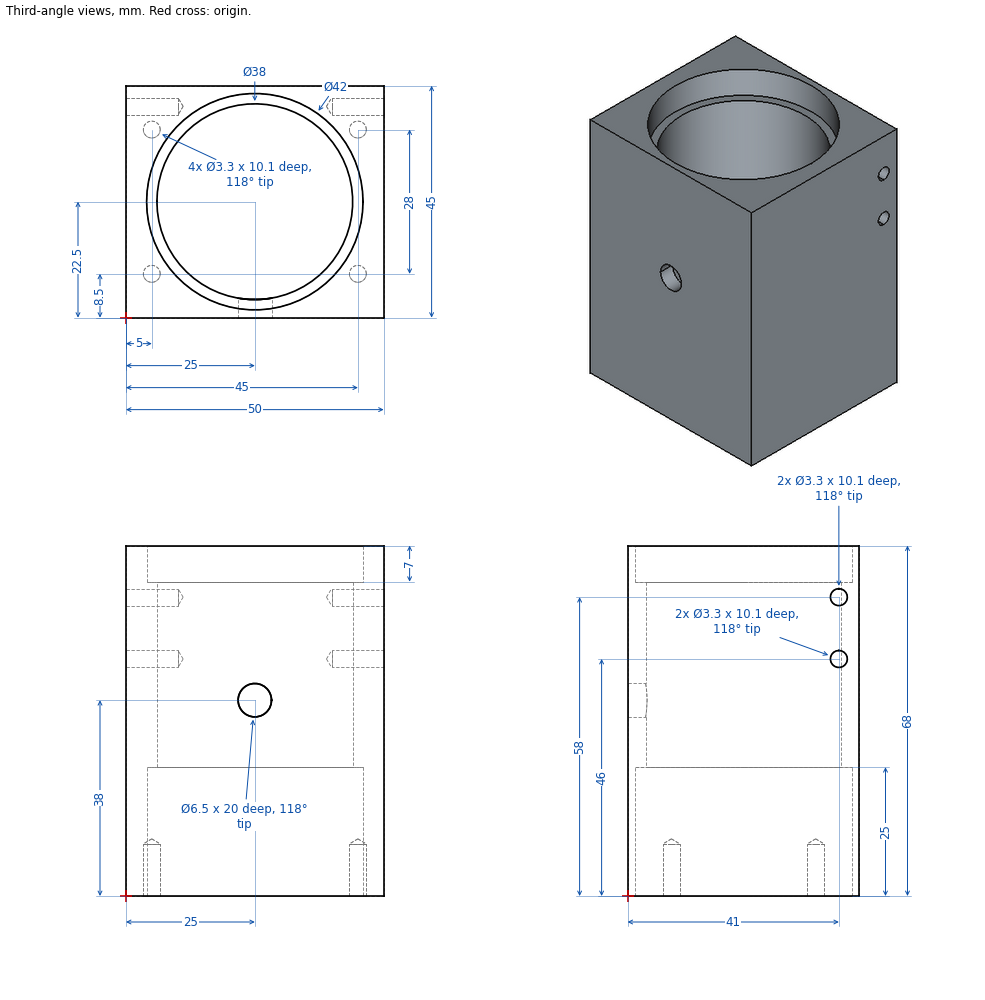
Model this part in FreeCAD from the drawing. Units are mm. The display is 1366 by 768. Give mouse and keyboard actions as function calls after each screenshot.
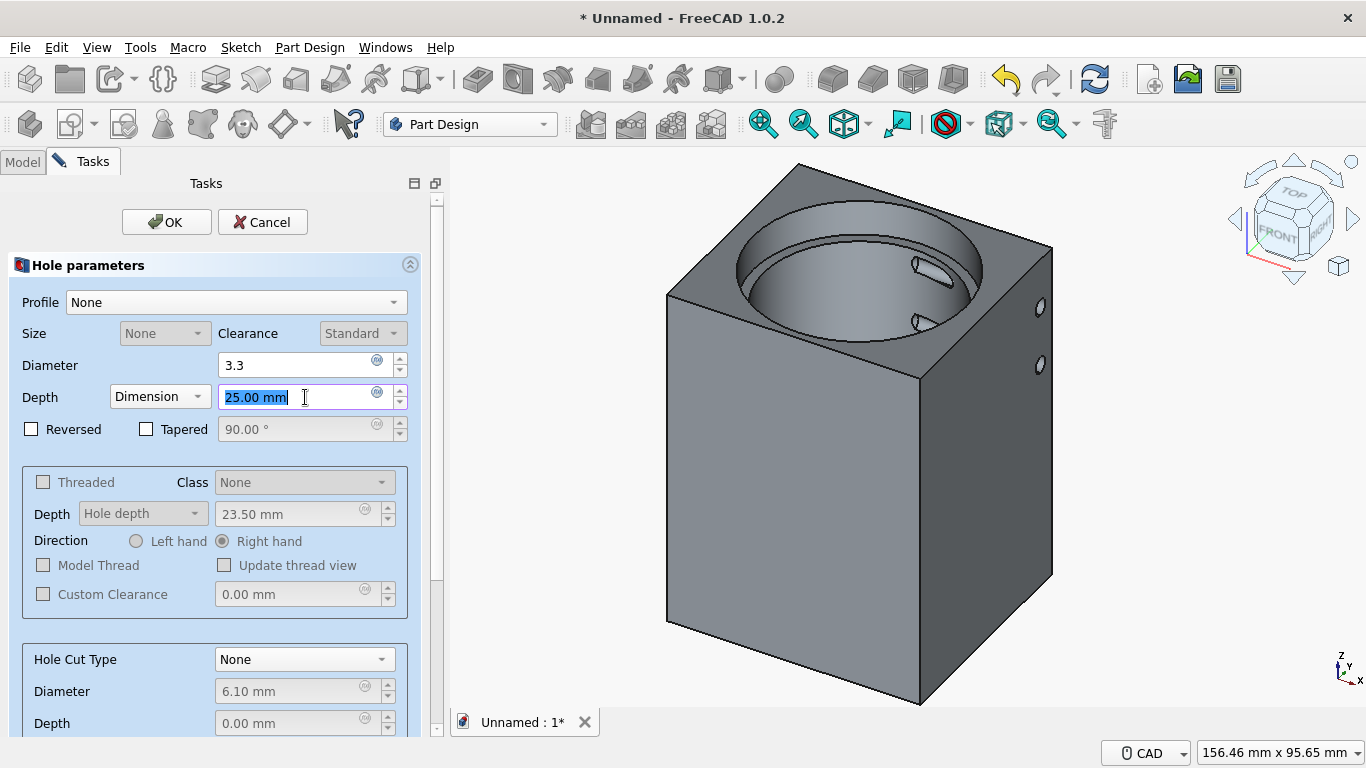
text(10.1)
key(Tab)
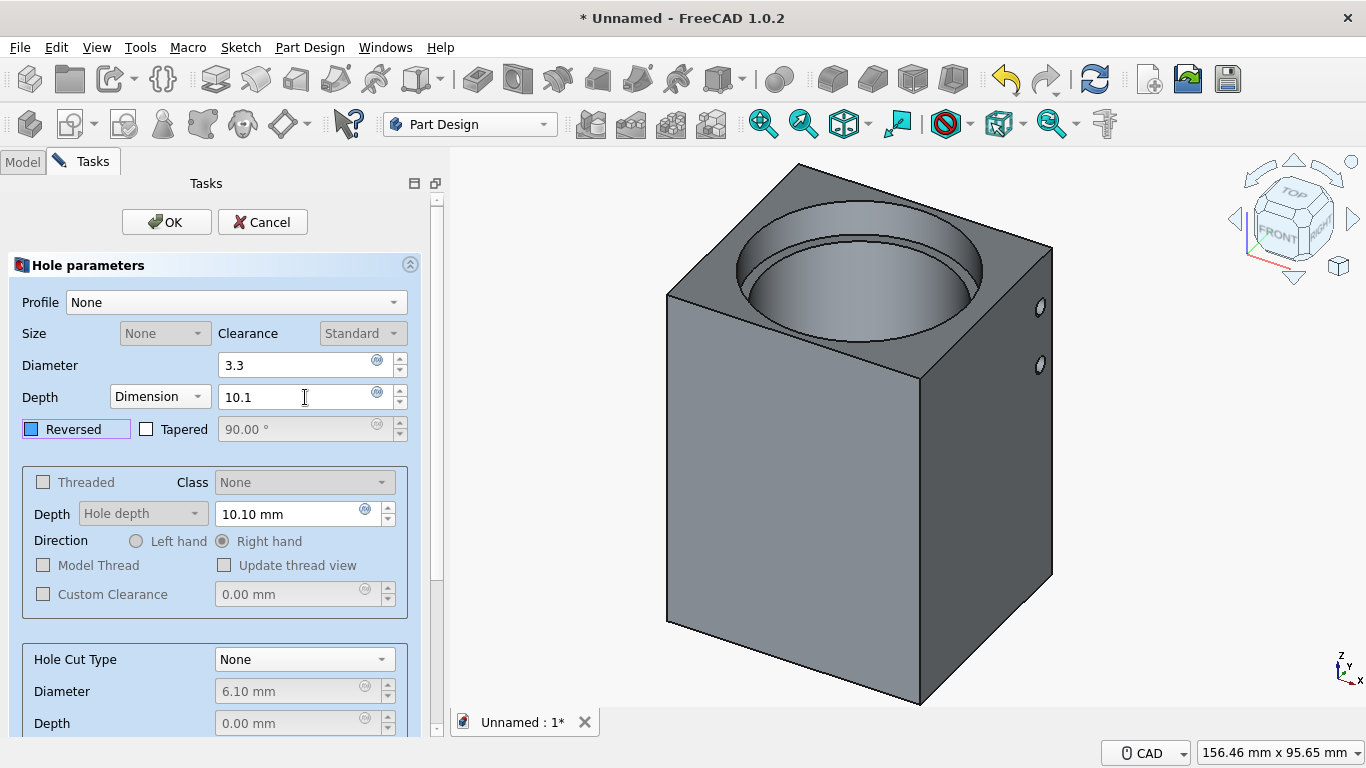
click(167, 222)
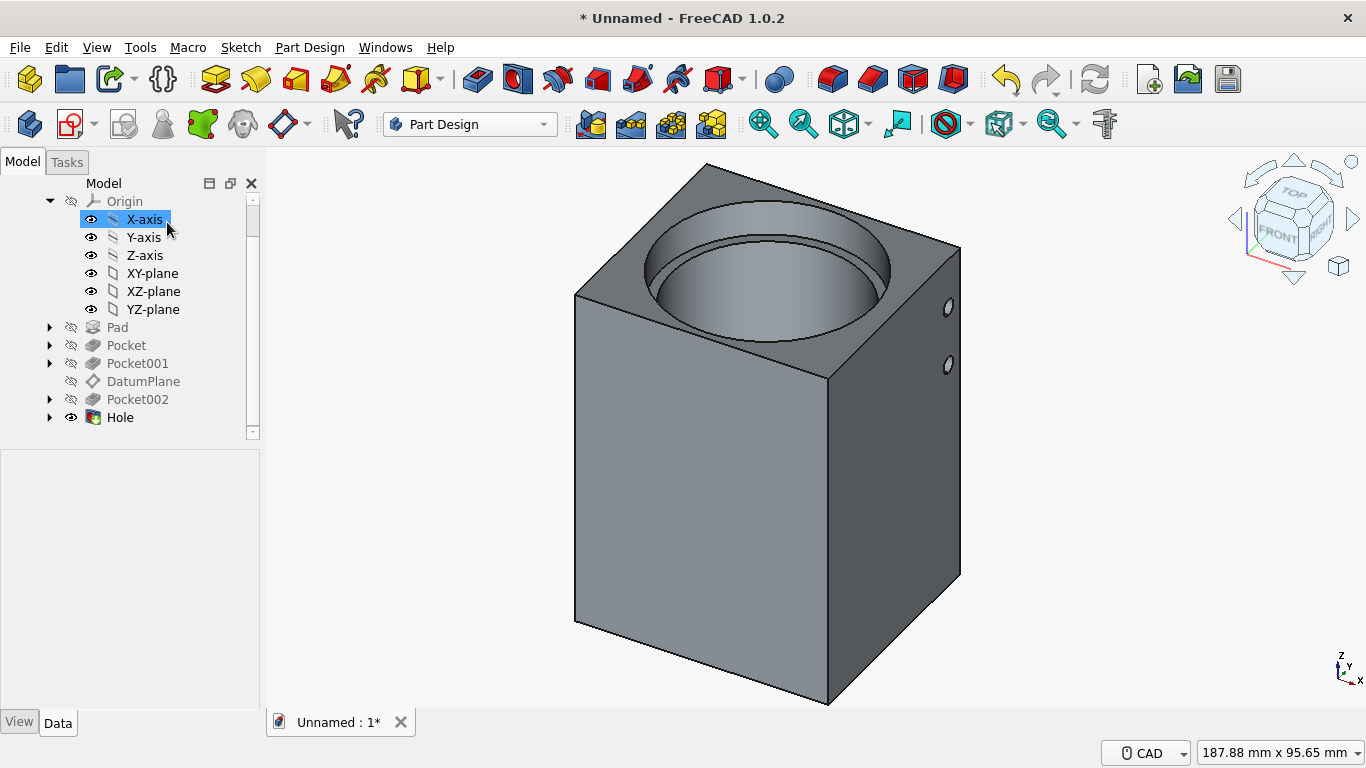
key(6)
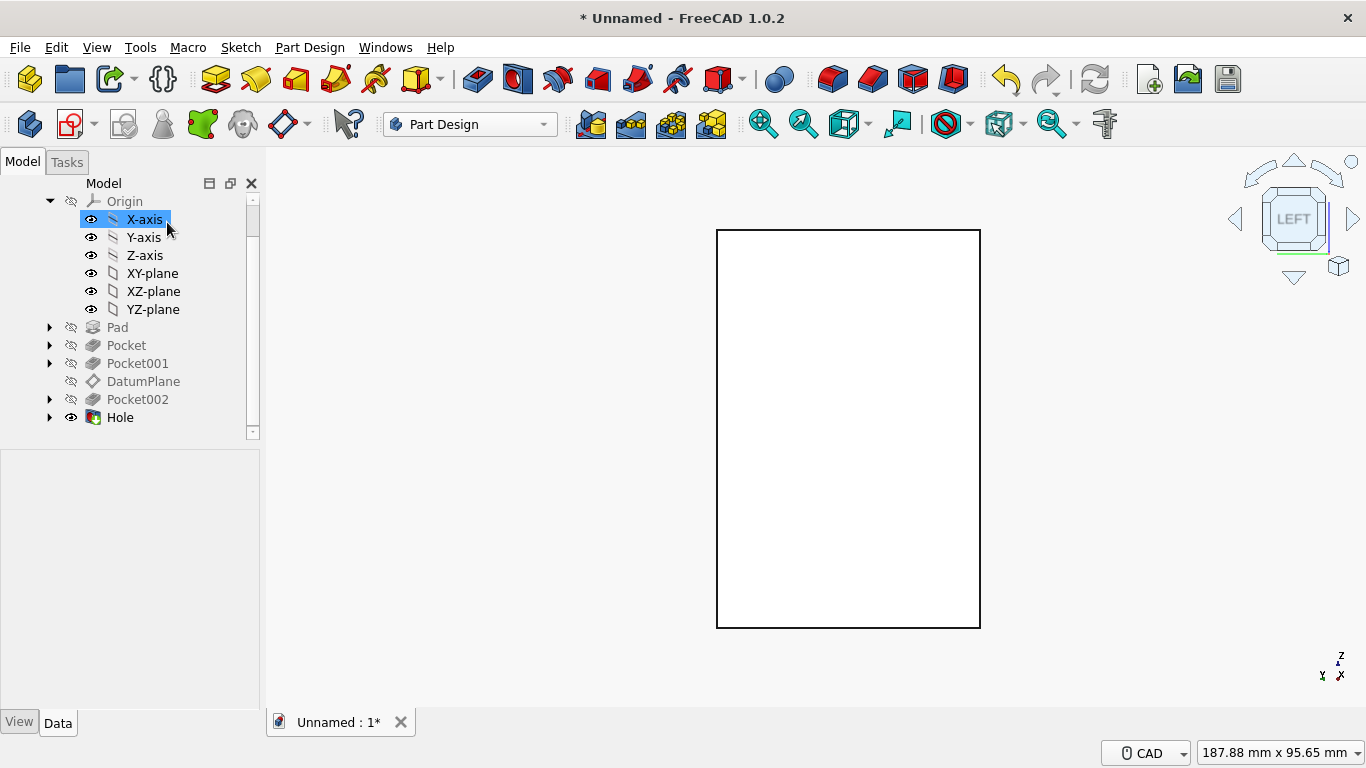
click(849, 372)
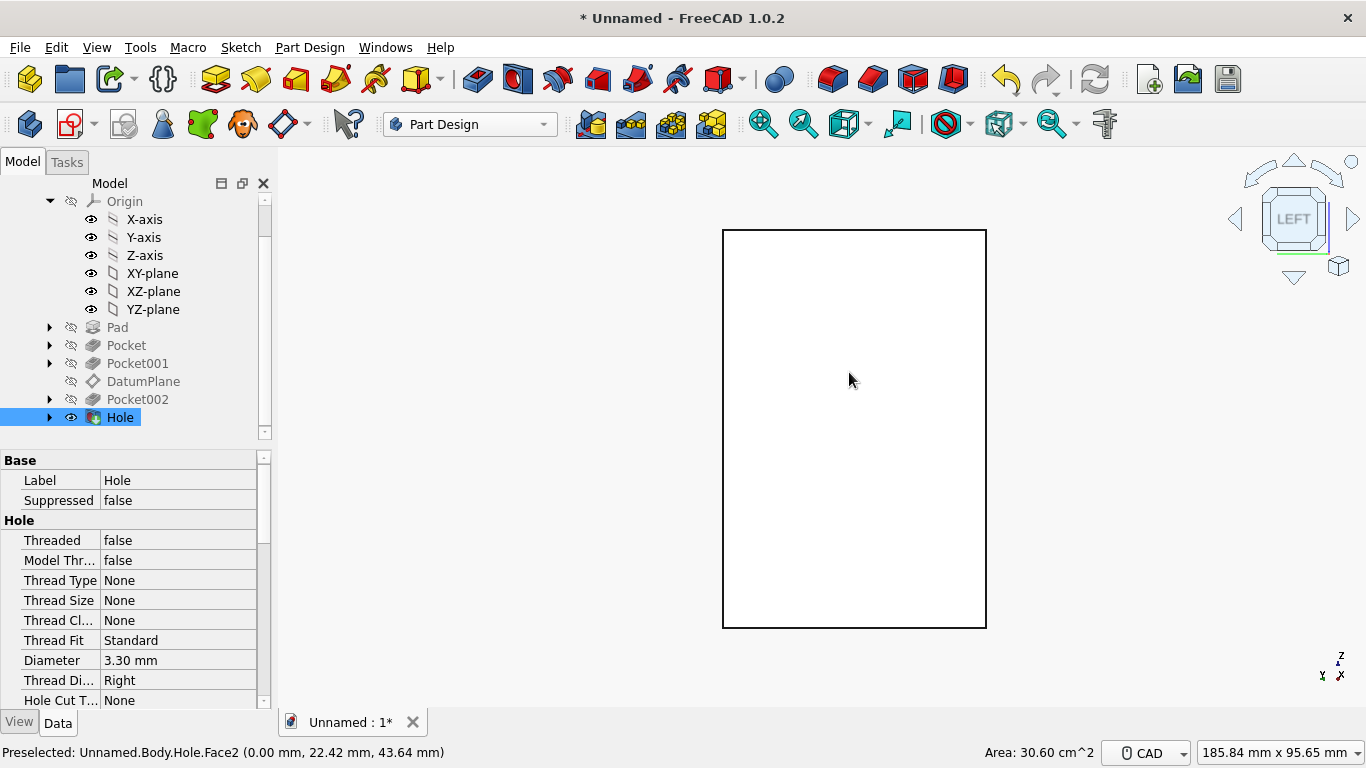
click(70, 124)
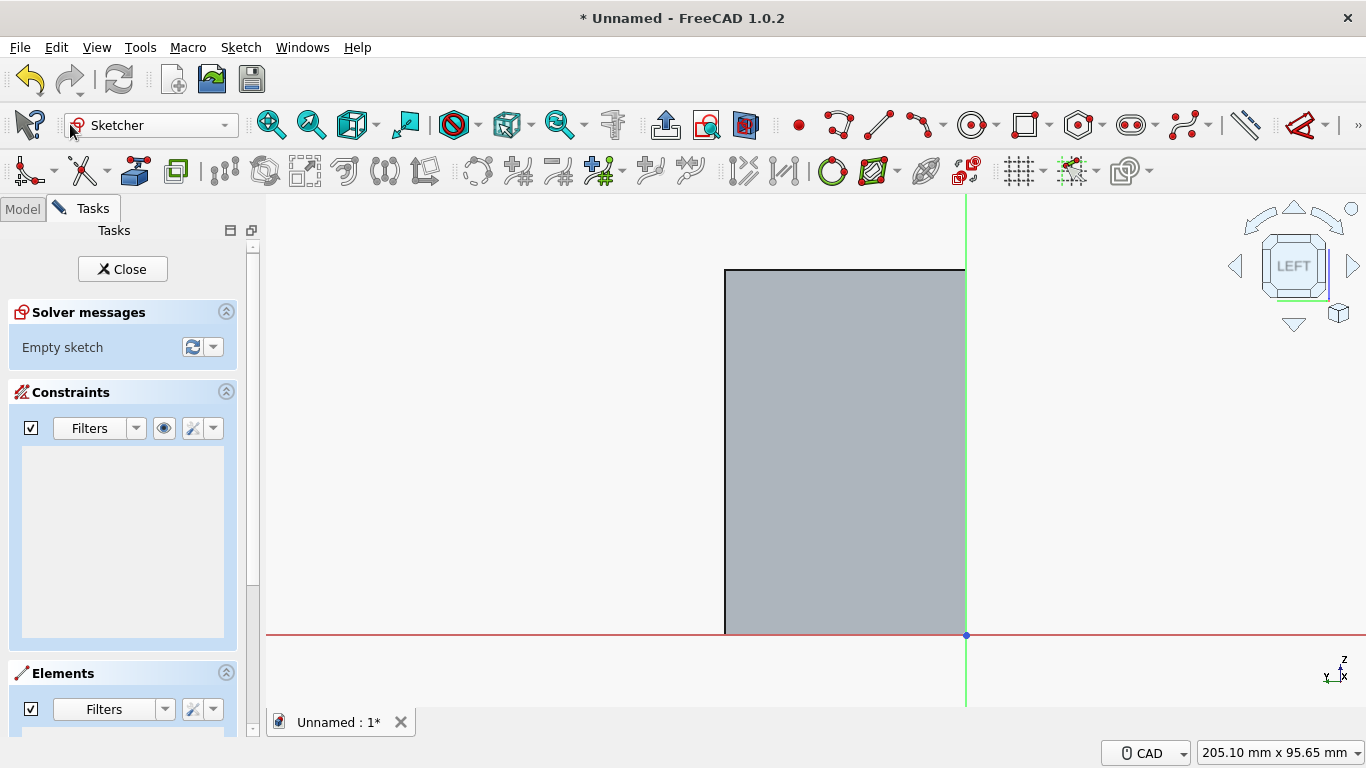
scroll(746, 325, up, 7)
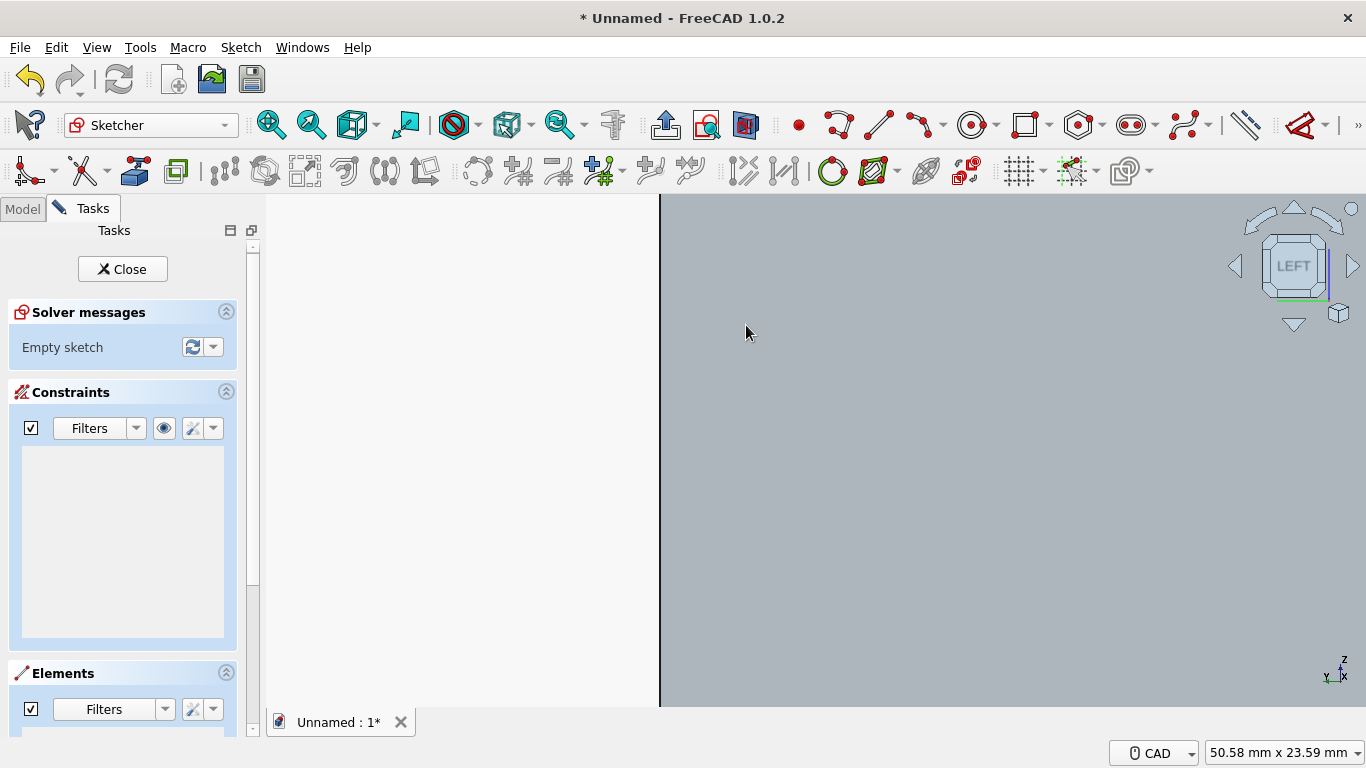
click(972, 126)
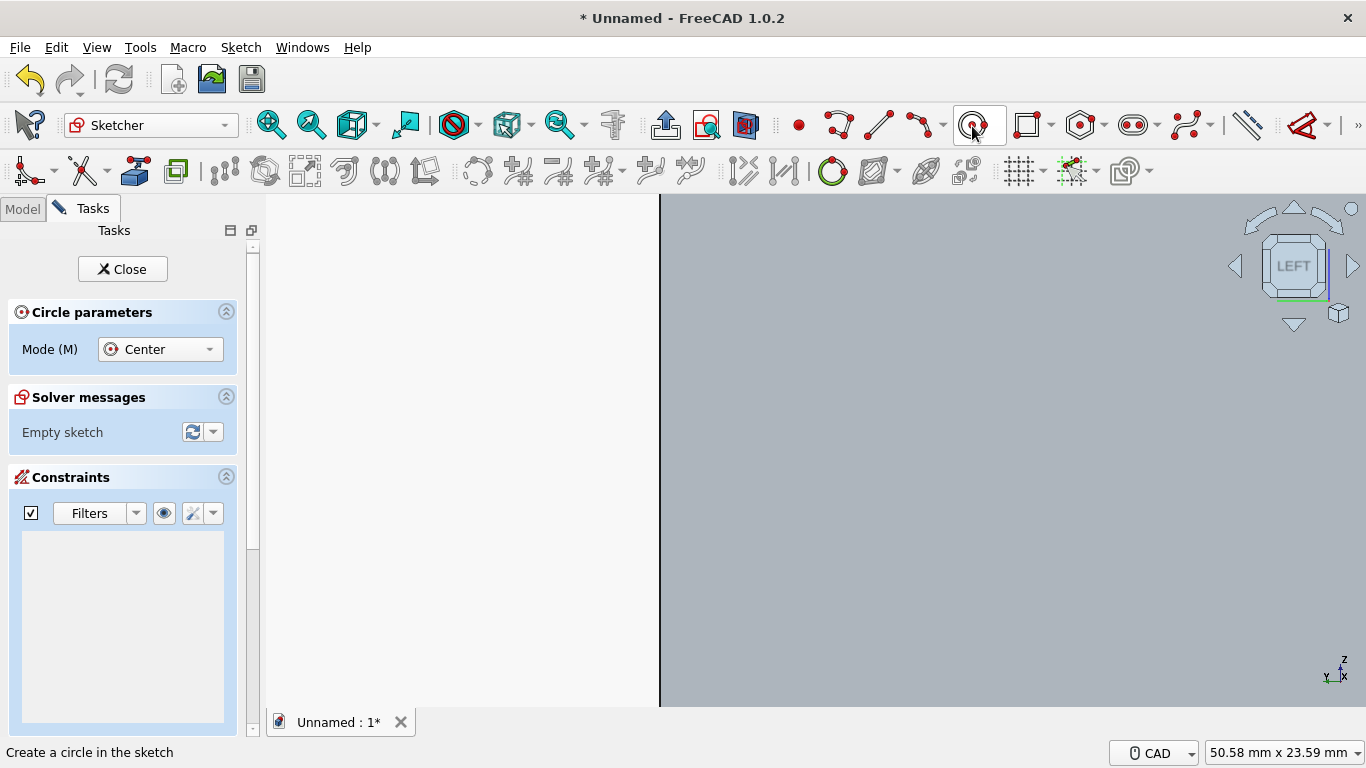
click(747, 581)
move(772, 556)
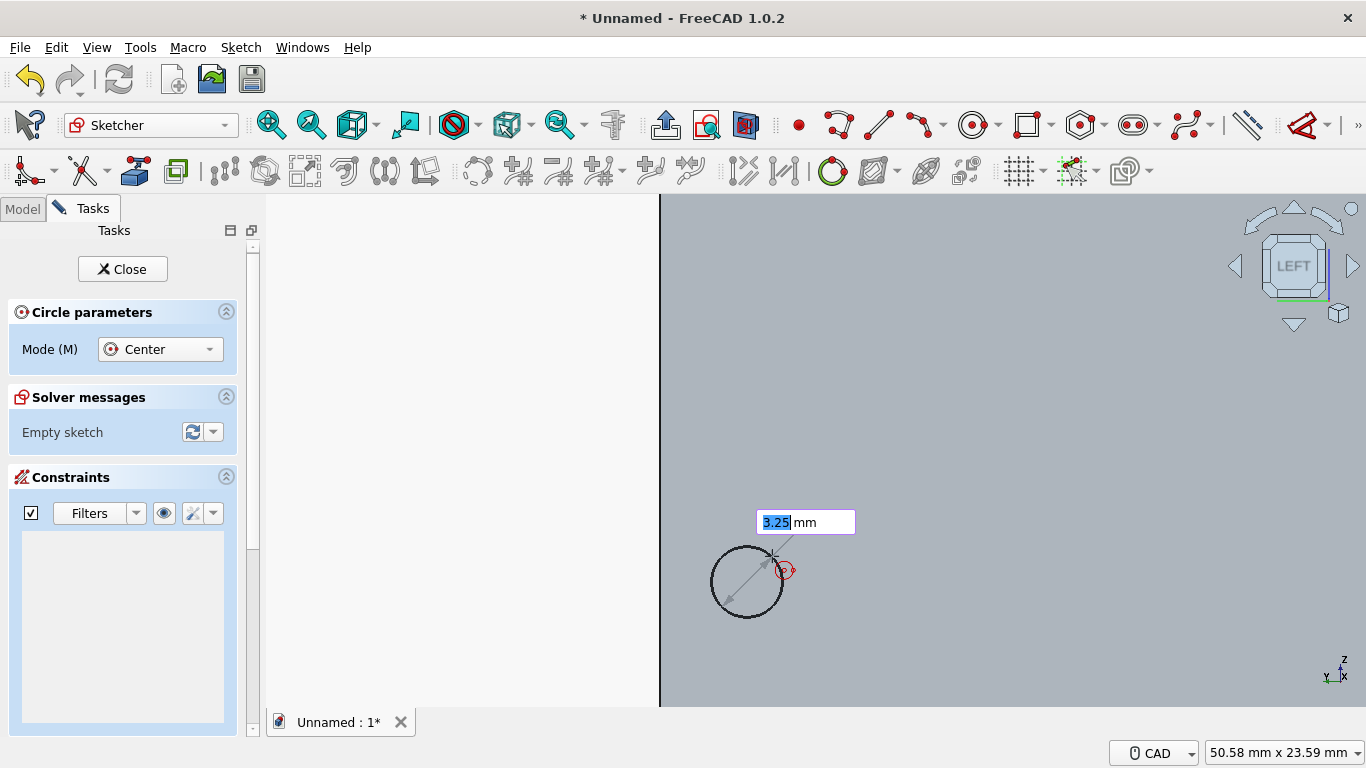
text(3.3)
key(Return)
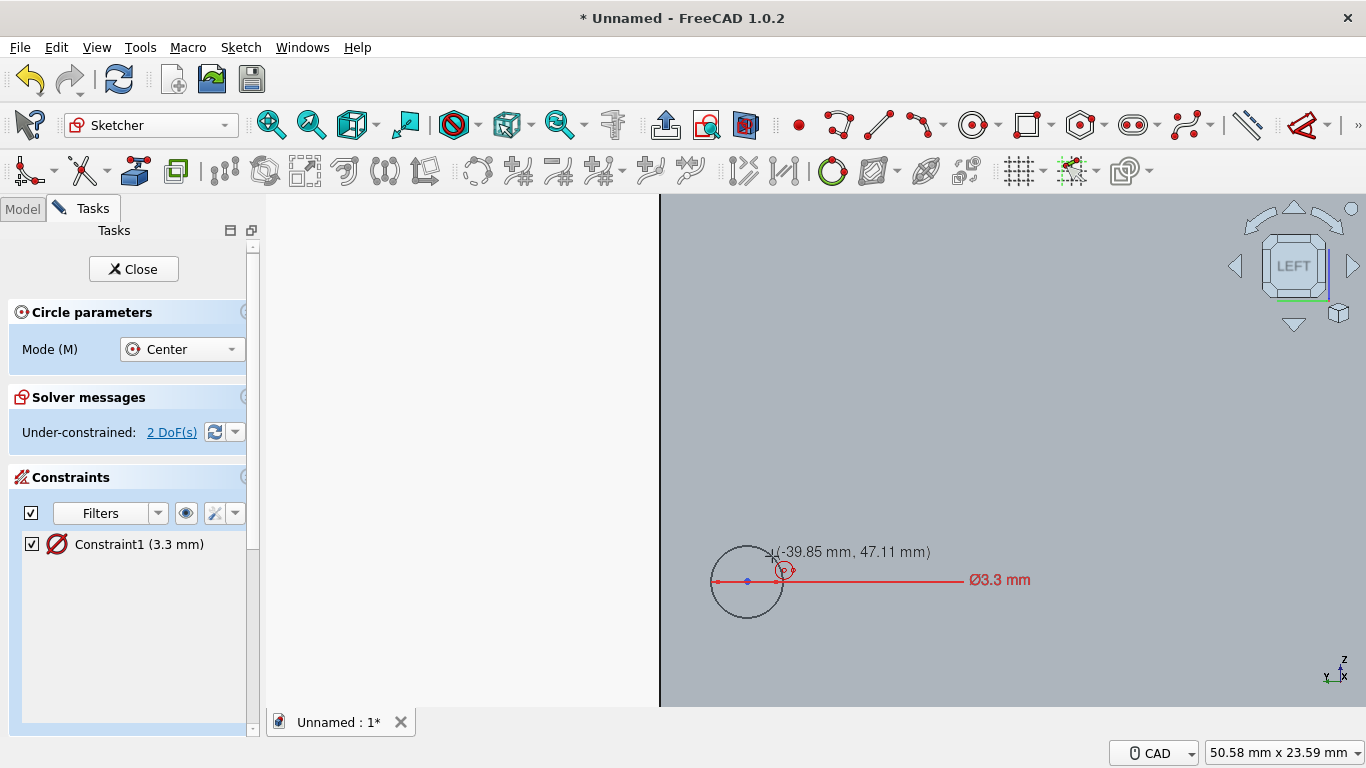
click(747, 320)
move(772, 295)